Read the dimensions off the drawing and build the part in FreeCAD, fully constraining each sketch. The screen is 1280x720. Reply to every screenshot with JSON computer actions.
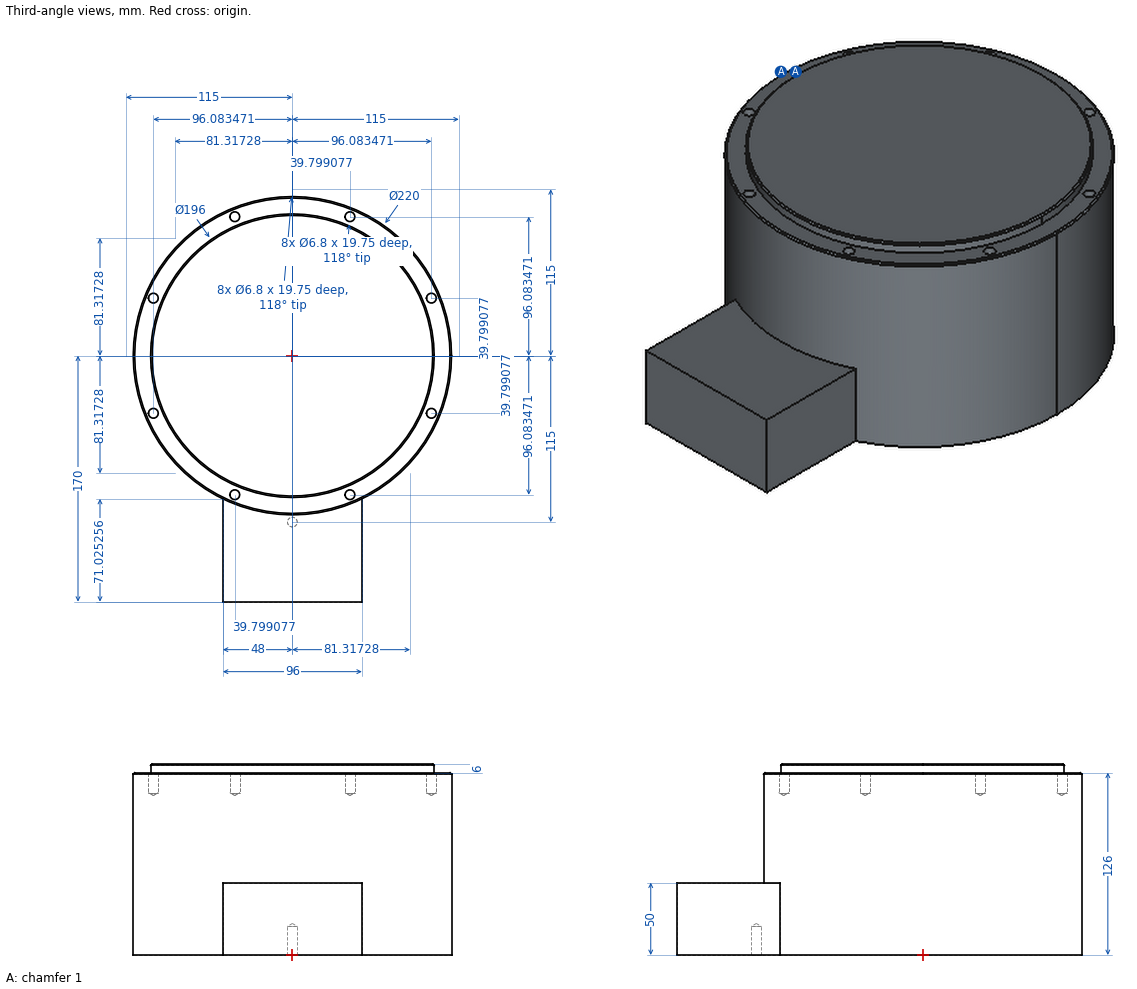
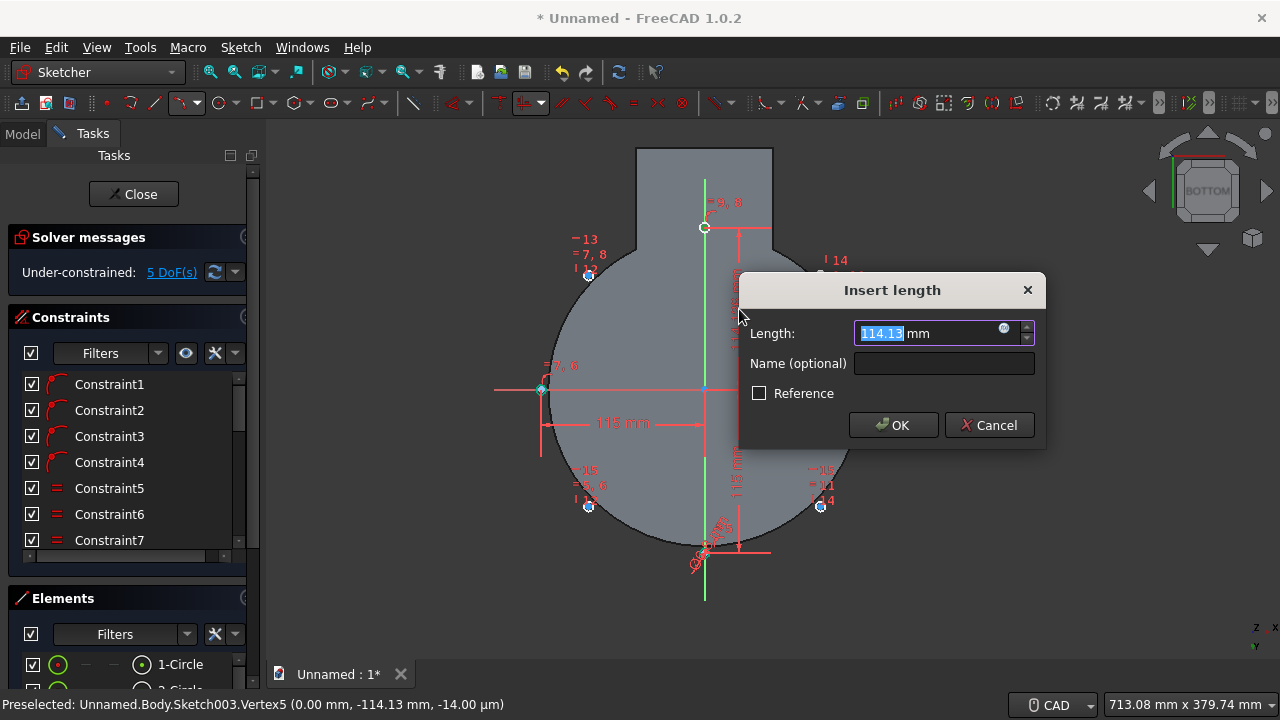
{"action": "type", "text": "115"}
{"action": "key", "text": "Return"}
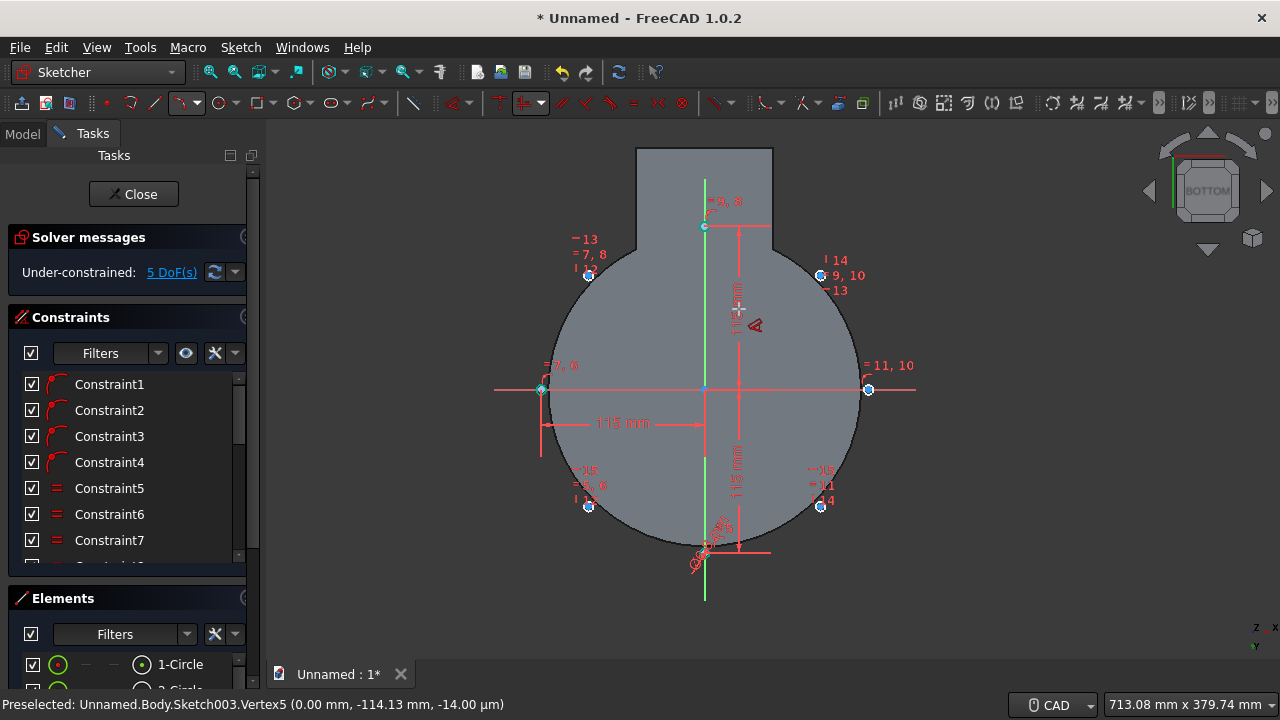
{"action": "left_click", "coordinate": [869, 390]}
{"action": "left_click", "coordinate": [787, 424]}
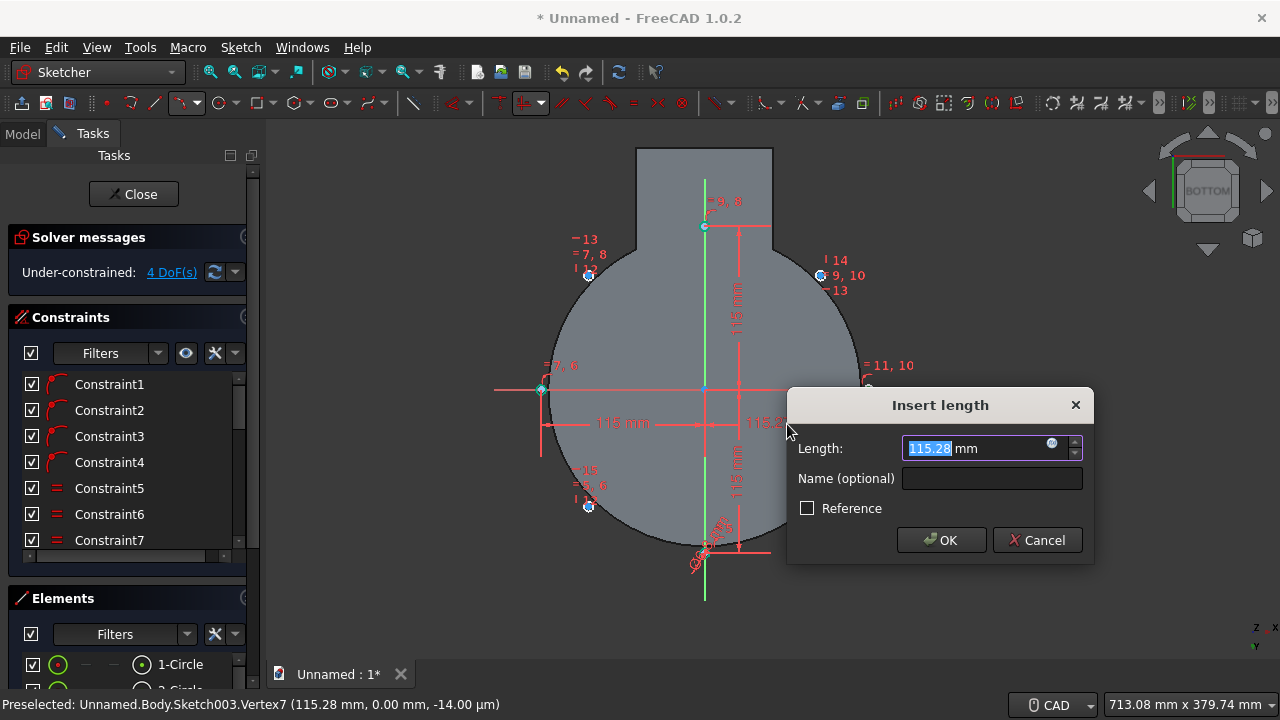
{"action": "type", "text": "115"}
{"action": "key", "text": "Return"}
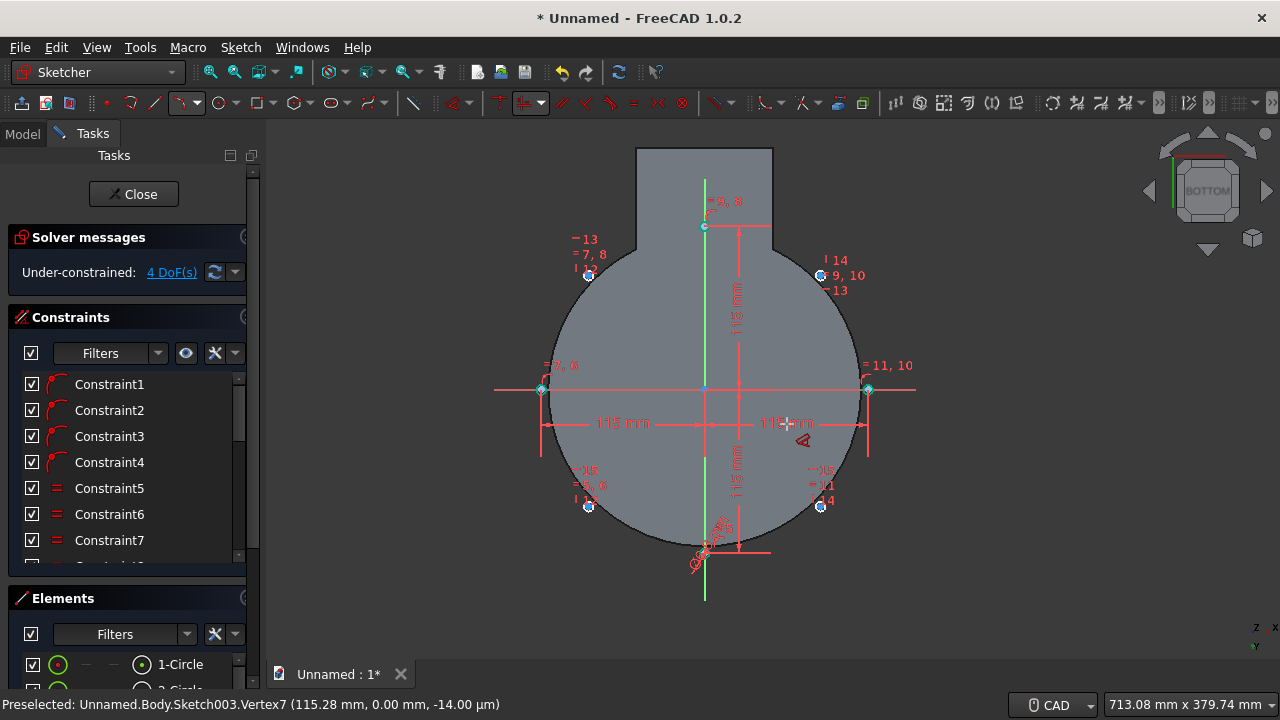
{"action": "left_click", "coordinate": [589, 507]}
{"action": "left_click", "coordinate": [620, 541]}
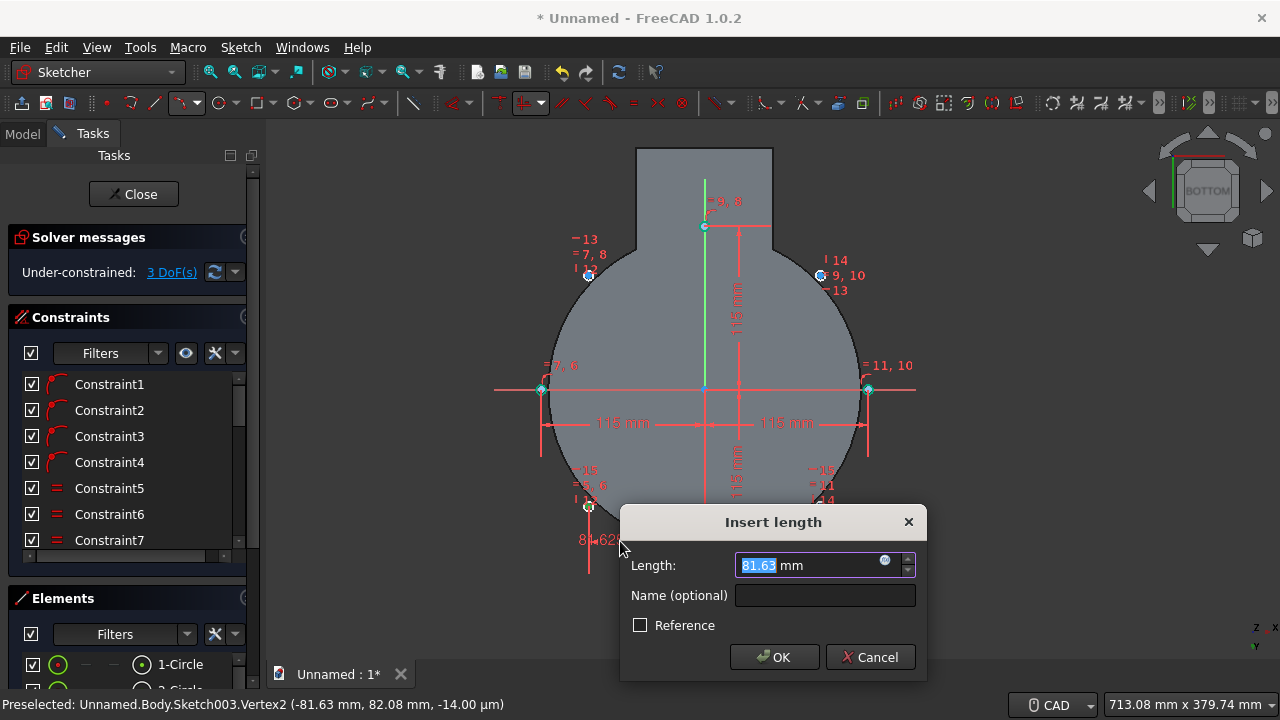
{"action": "type", "text": "81.31728"}
{"action": "key", "text": "Return"}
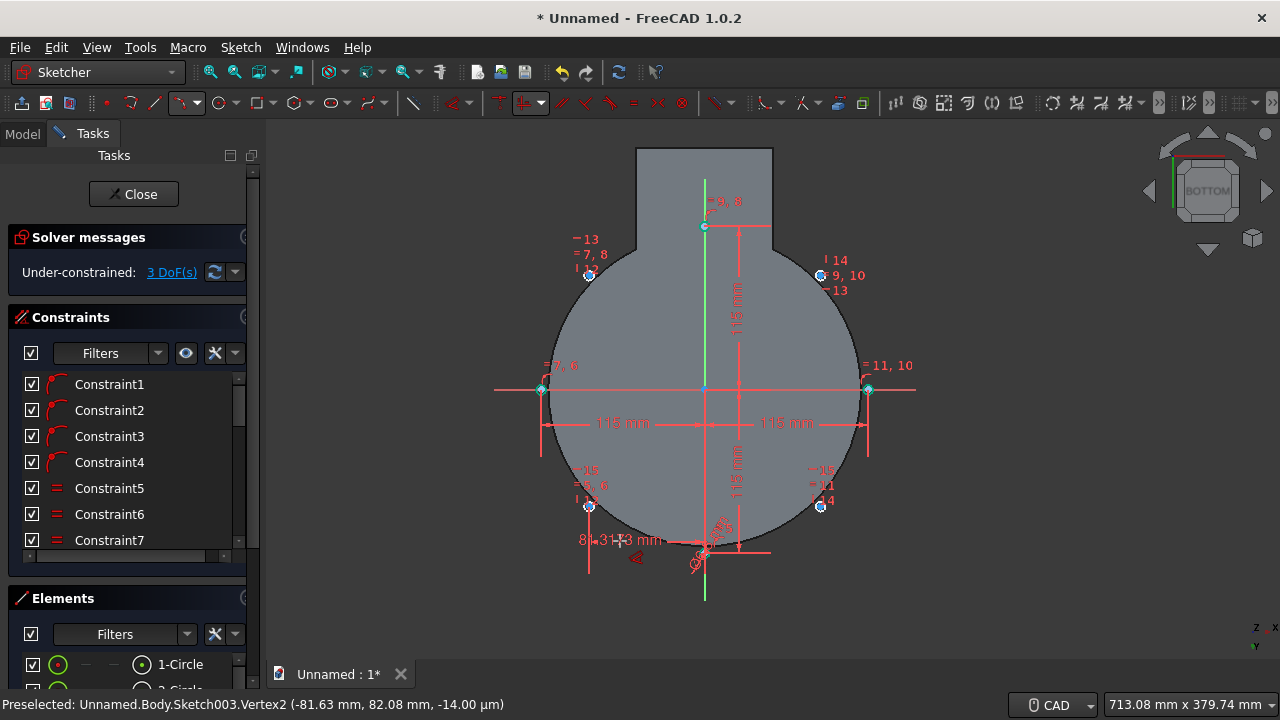
{"action": "left_click", "coordinate": [589, 507]}
{"action": "left_click", "coordinate": [555, 448]}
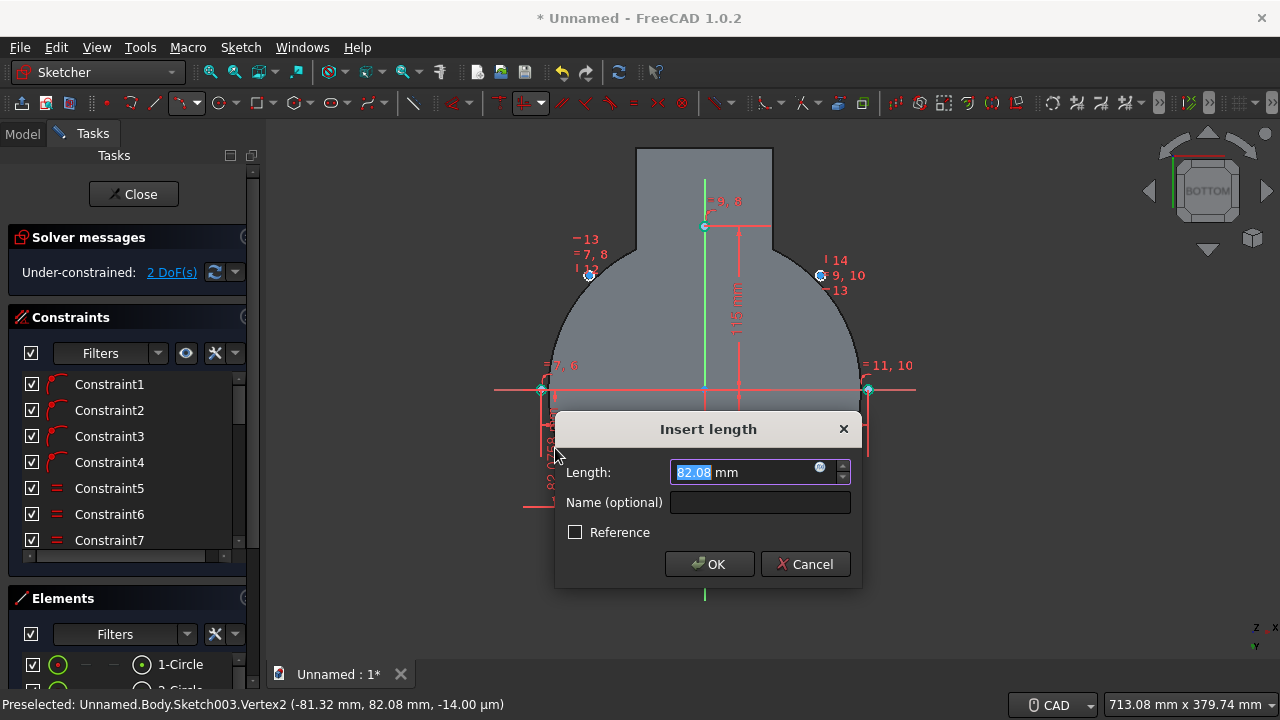
{"action": "type", "text": "81.31728"}
{"action": "key", "text": "Return"}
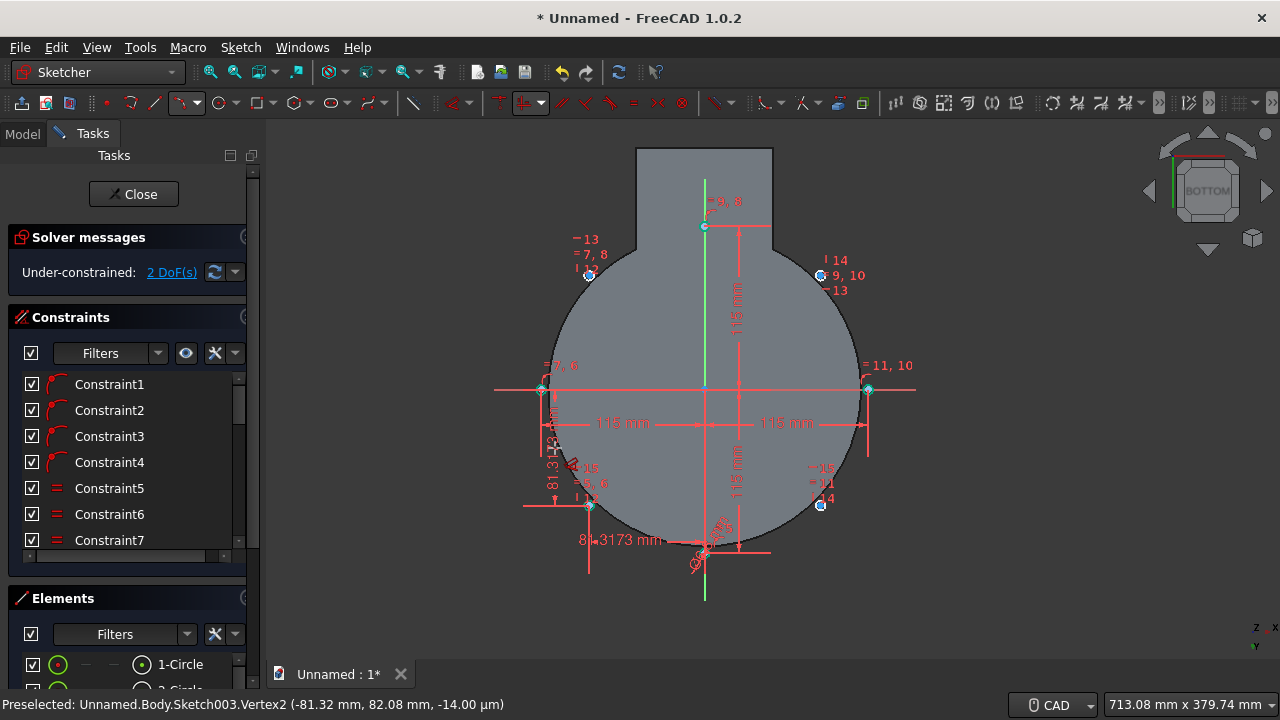
{"action": "left_click", "coordinate": [589, 276]}
{"action": "left_click", "coordinate": [555, 333]}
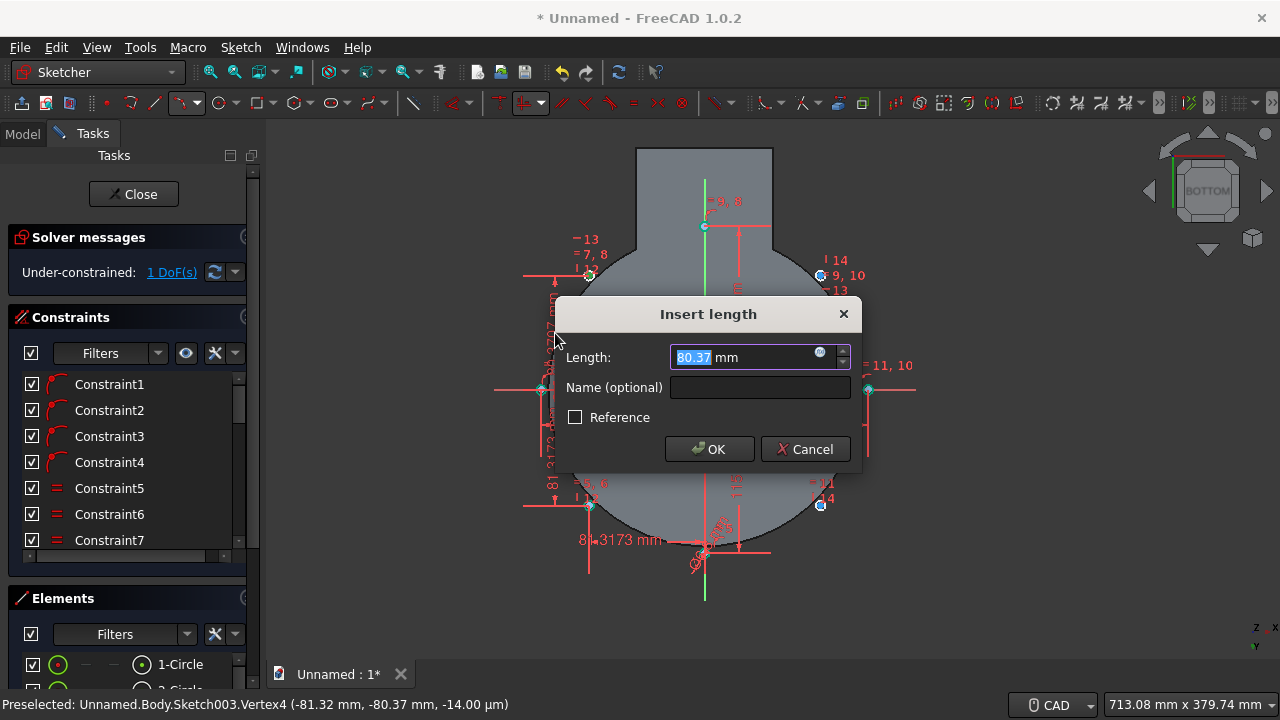
{"action": "type", "text": "81.31728"}
{"action": "key", "text": "Return"}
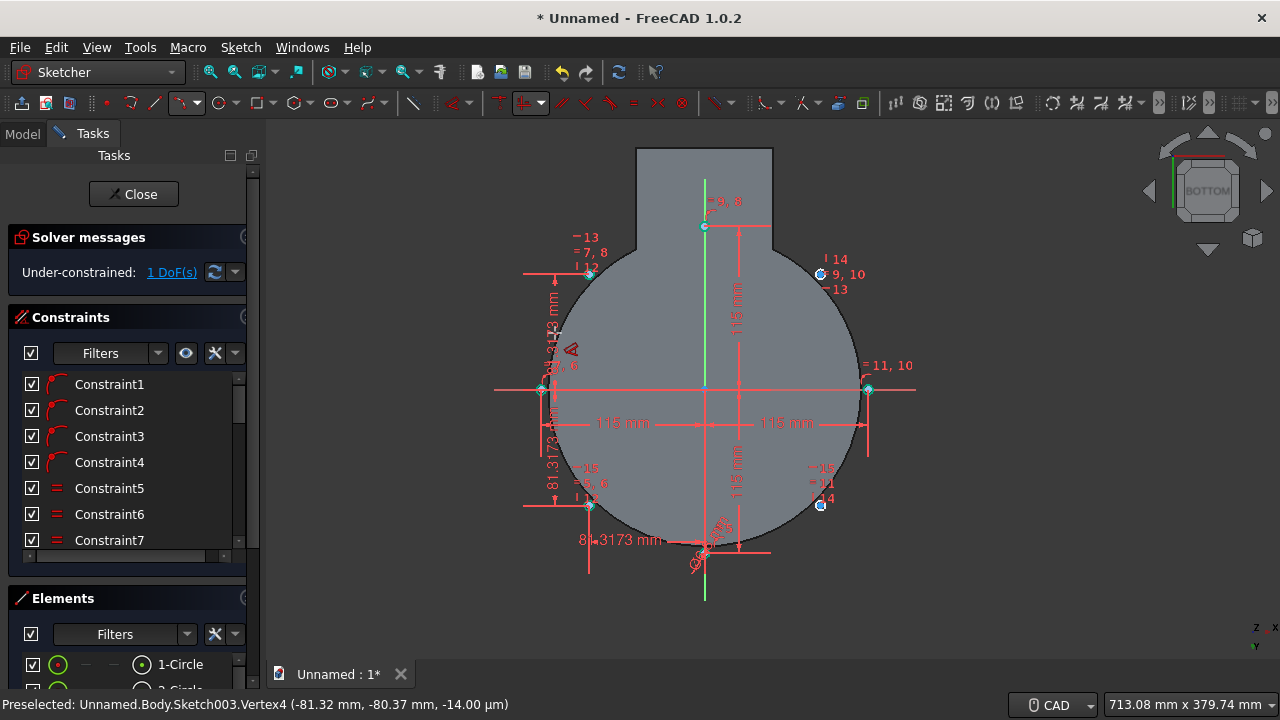
{"action": "left_click", "coordinate": [821, 274]}
{"action": "left_click", "coordinate": [763, 240]}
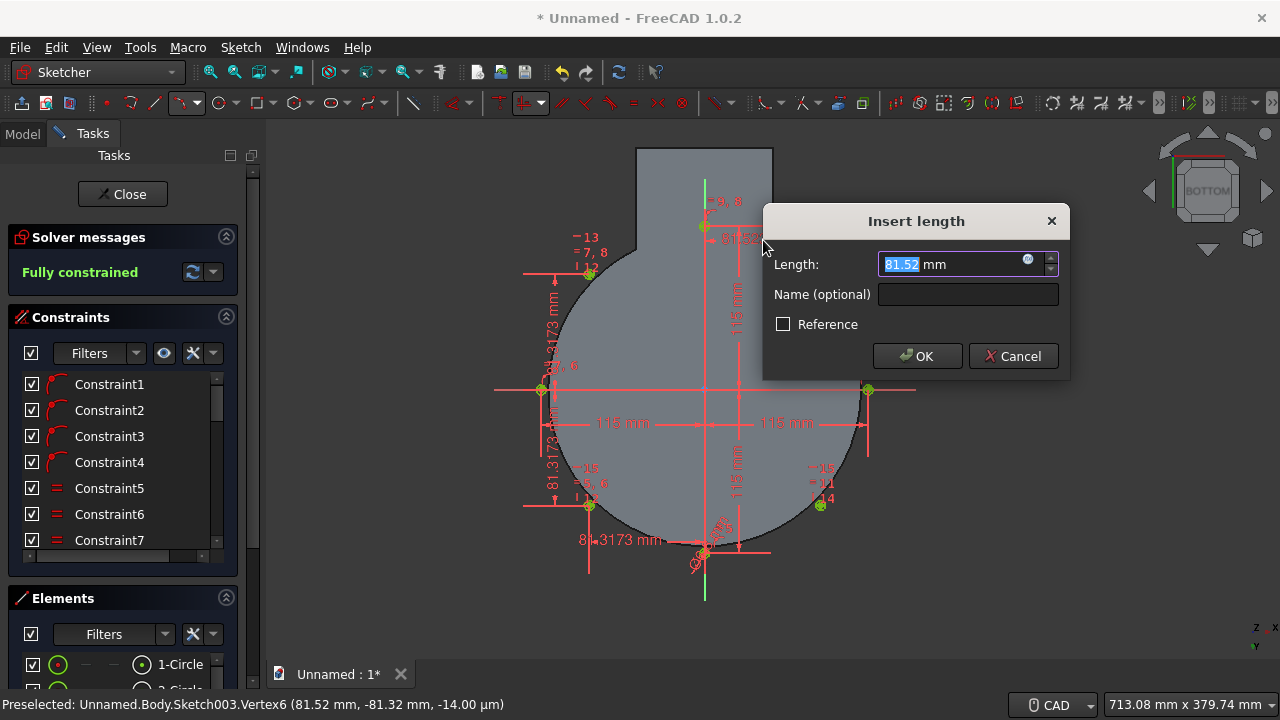
{"action": "type", "text": "81.31728"}
{"action": "key", "text": "Return"}
{"action": "key", "text": "Escape"}